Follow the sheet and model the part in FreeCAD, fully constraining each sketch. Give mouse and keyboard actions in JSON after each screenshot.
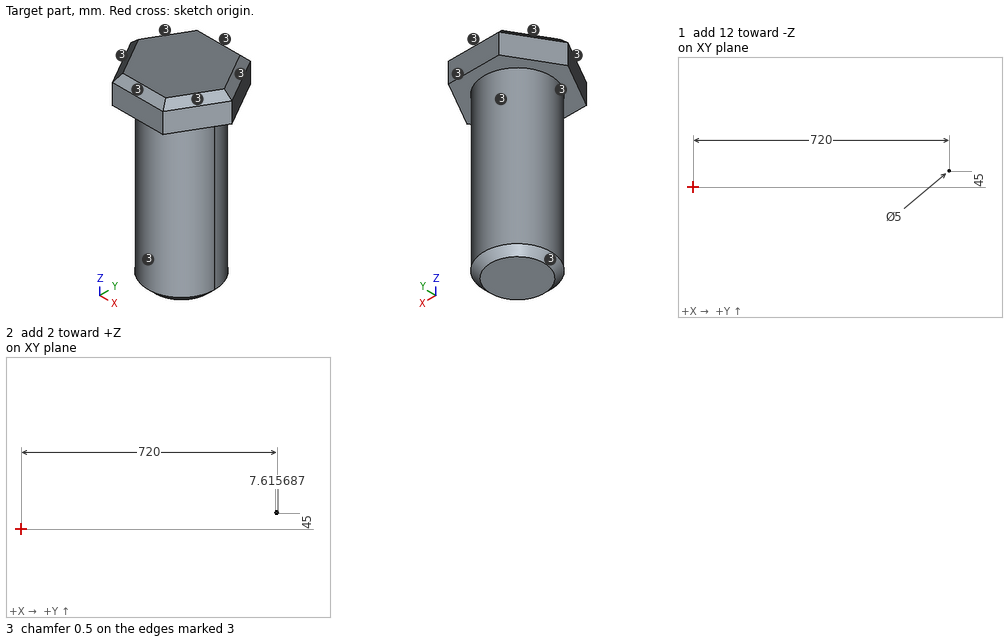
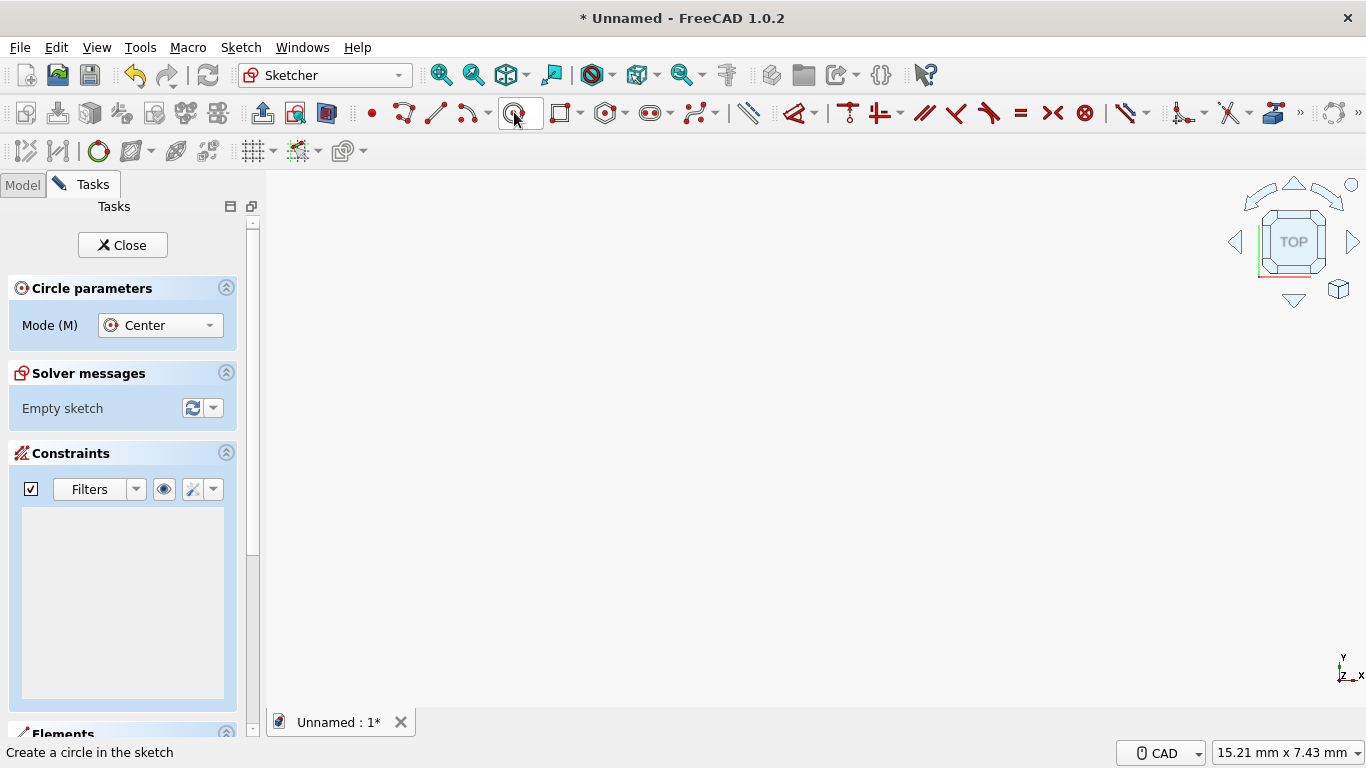
{"action": "left_click", "coordinate": [744, 437]}
{"action": "left_click", "coordinate": [871, 309]}
{"action": "key", "text": "Escape"}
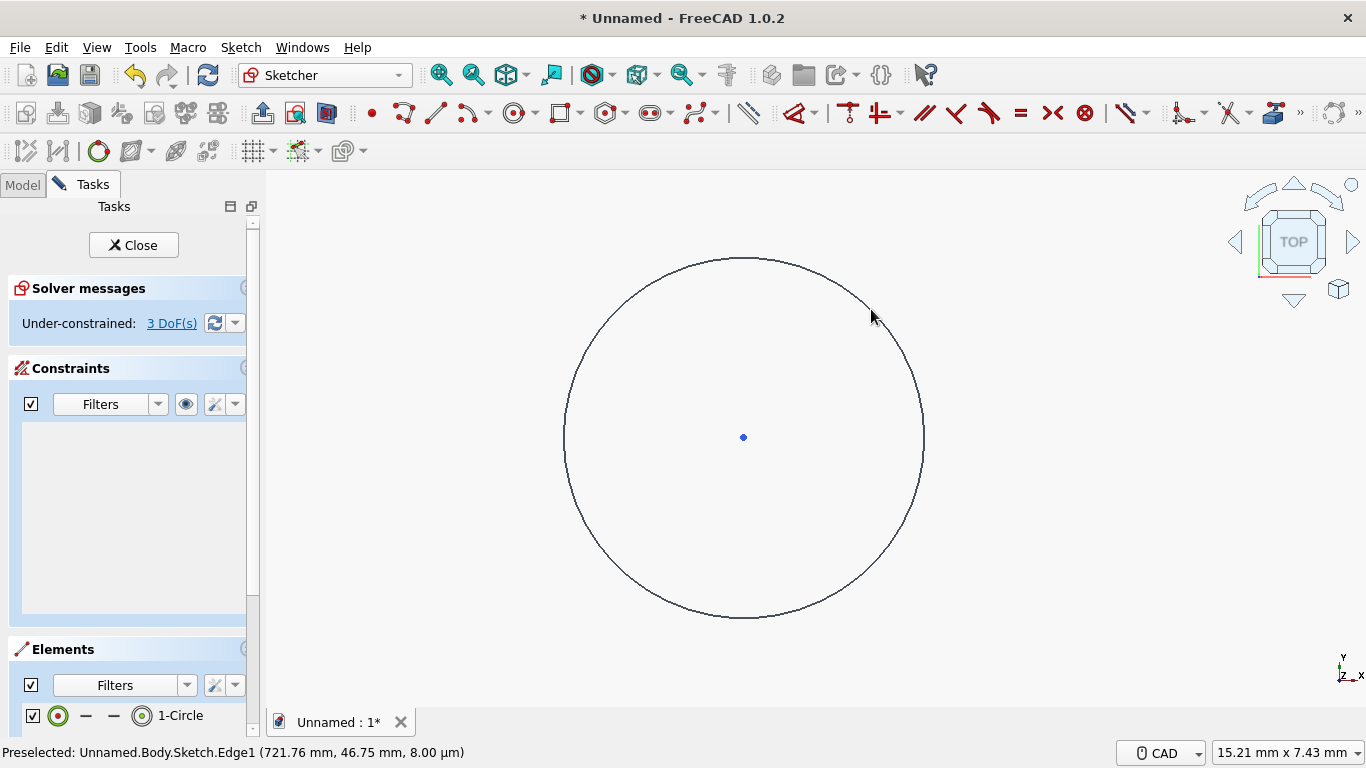
{"action": "key", "text": "d"}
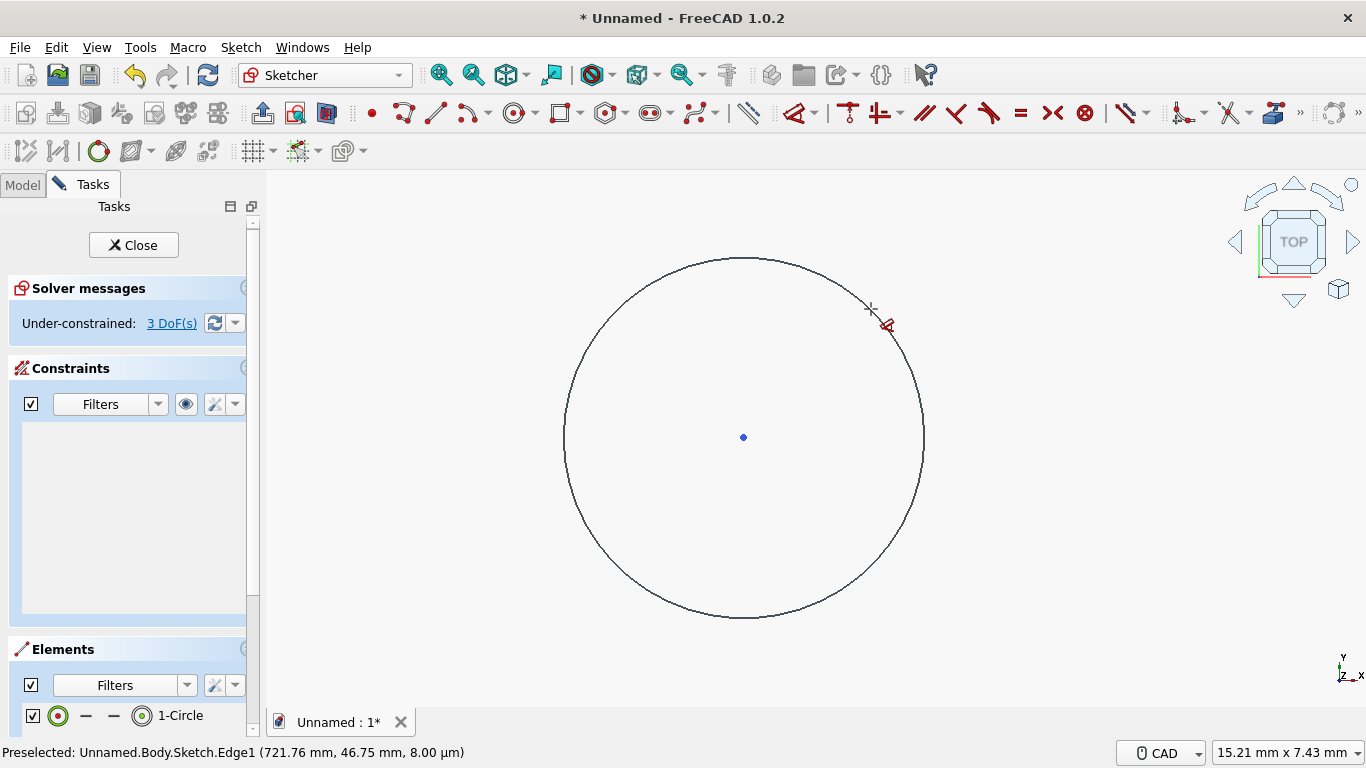
{"action": "left_click", "coordinate": [871, 310]}
{"action": "left_click", "coordinate": [894, 287]}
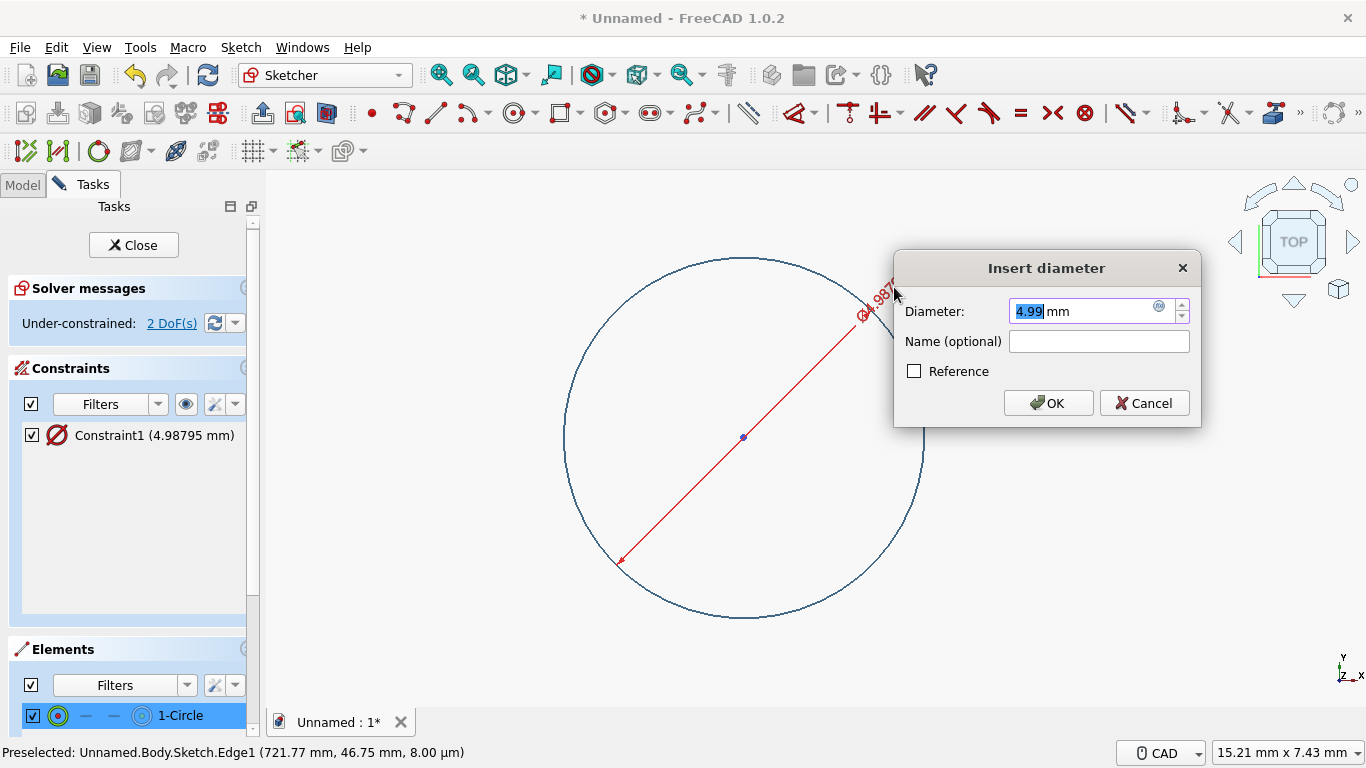
{"action": "type", "text": "5"}
{"action": "key", "text": "Return"}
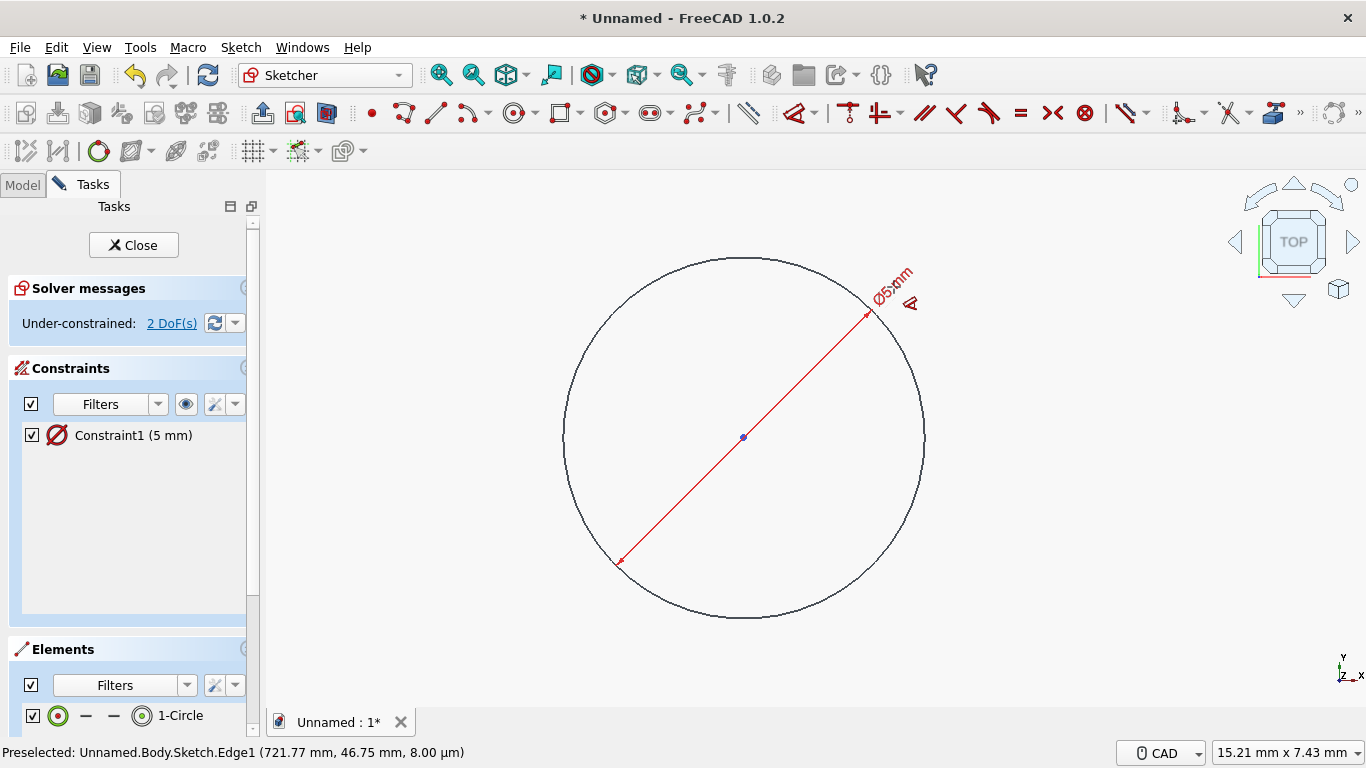
{"action": "left_click", "coordinate": [744, 438]}
{"action": "left_click", "coordinate": [778, 558]}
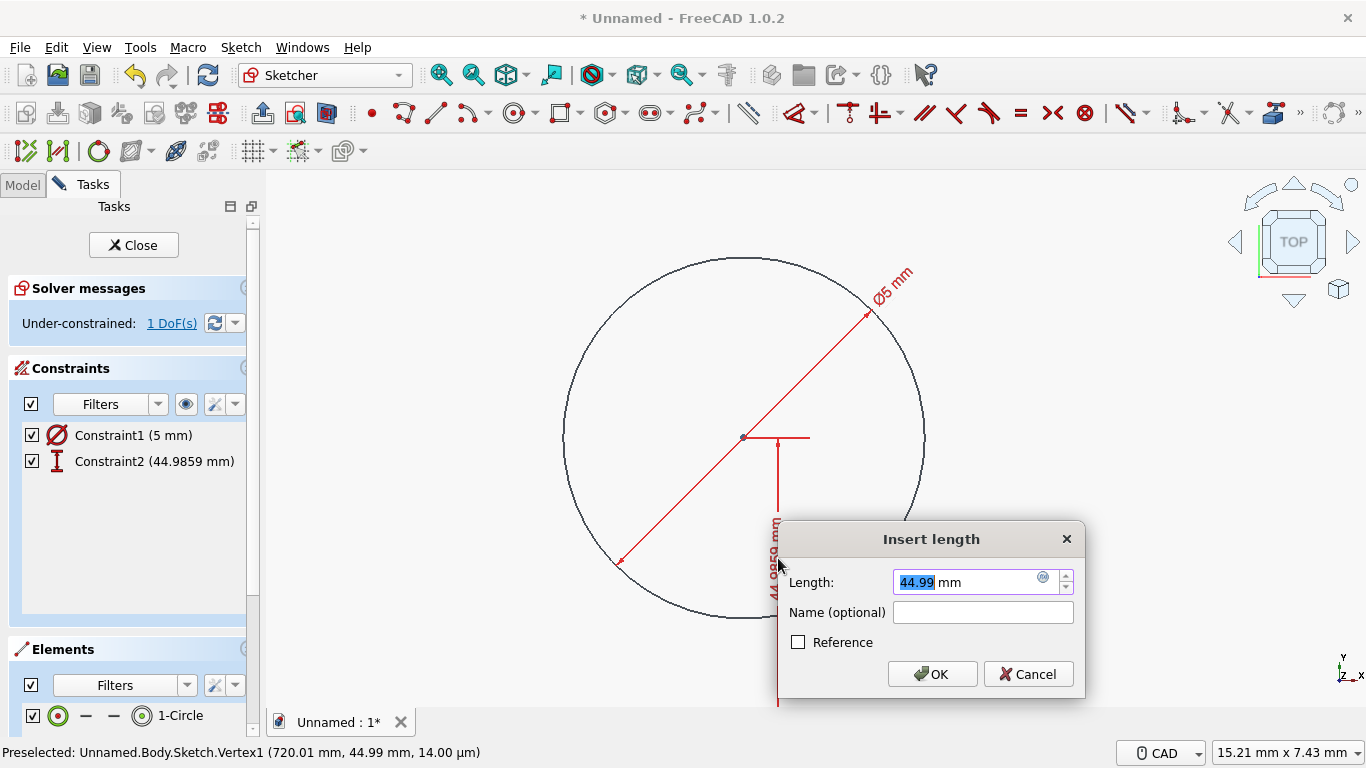
{"action": "type", "text": "45"}
{"action": "key", "text": "Return"}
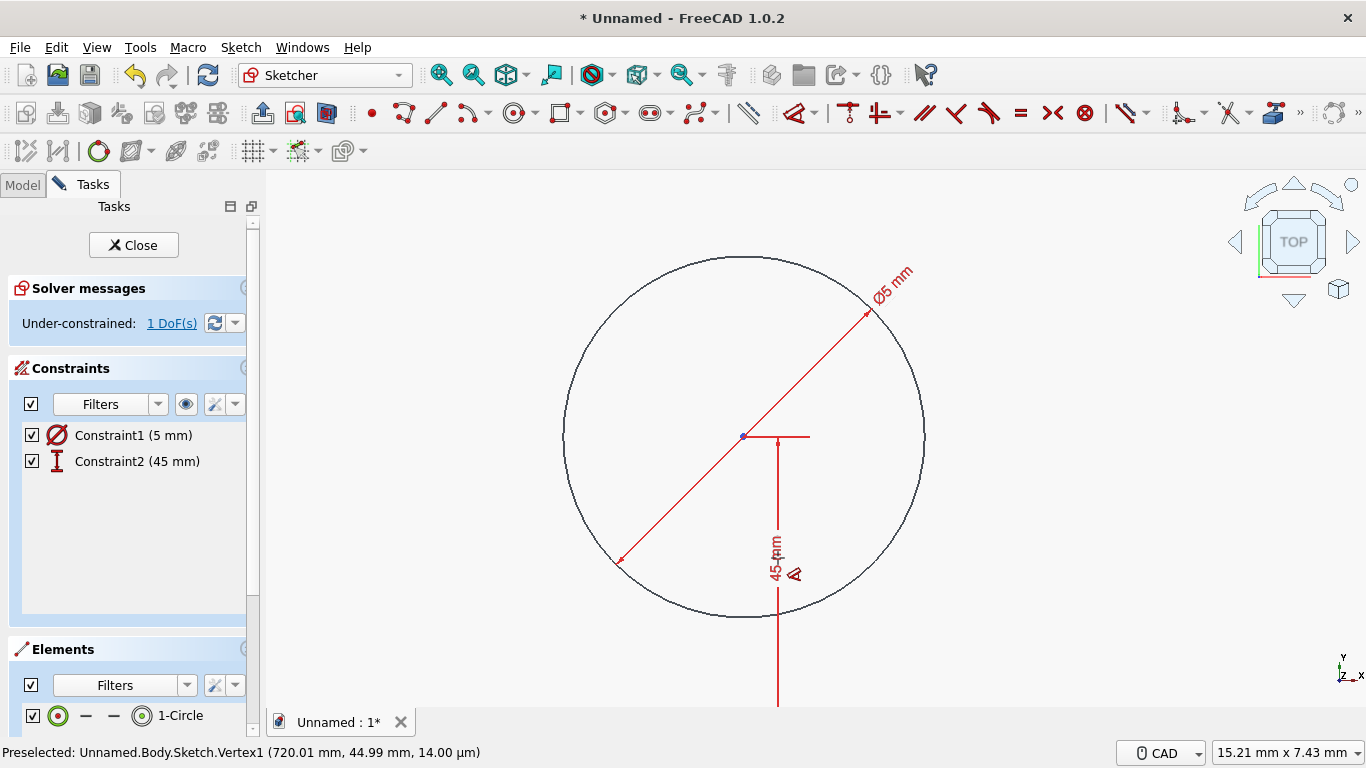
{"action": "left_click", "coordinate": [744, 437]}
{"action": "left_click", "coordinate": [519, 403]}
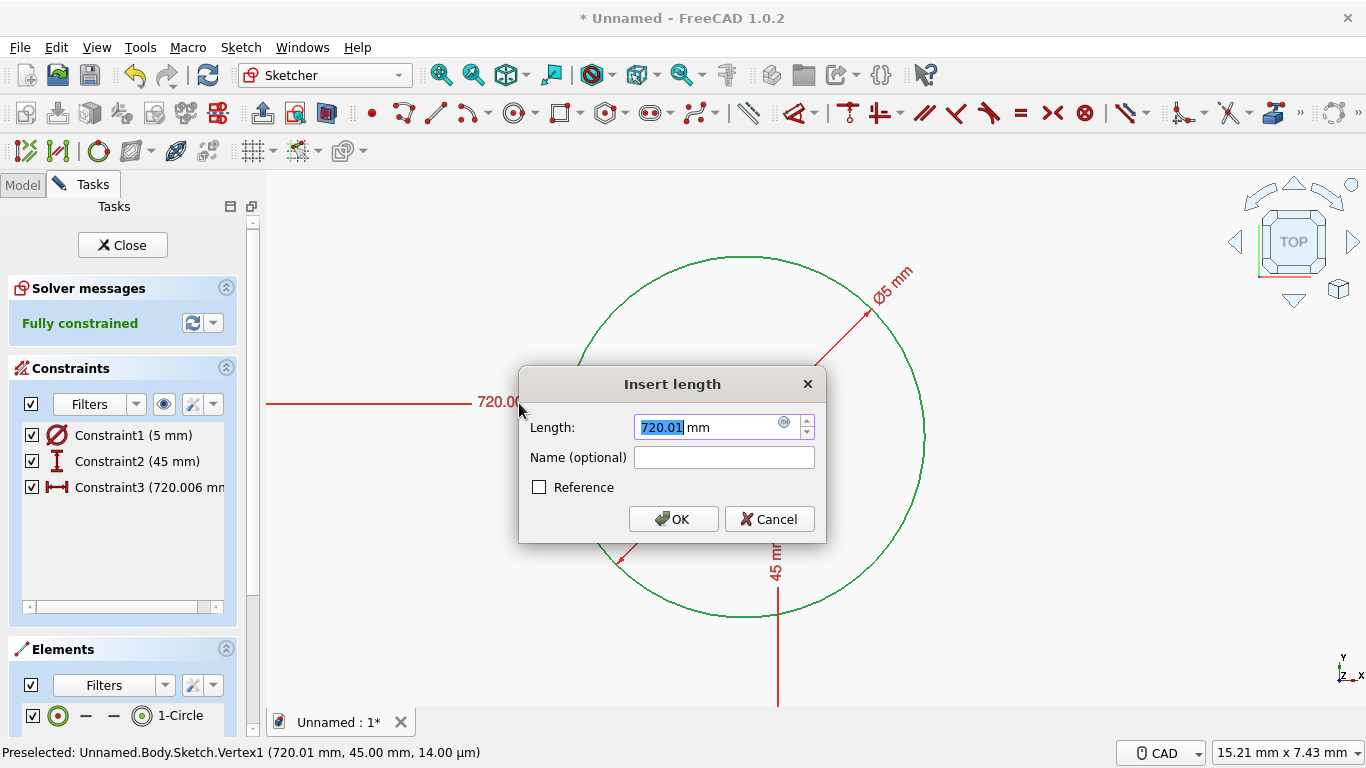
{"action": "type", "text": "720"}
{"action": "key", "text": "Return"}
{"action": "key", "text": "Escape"}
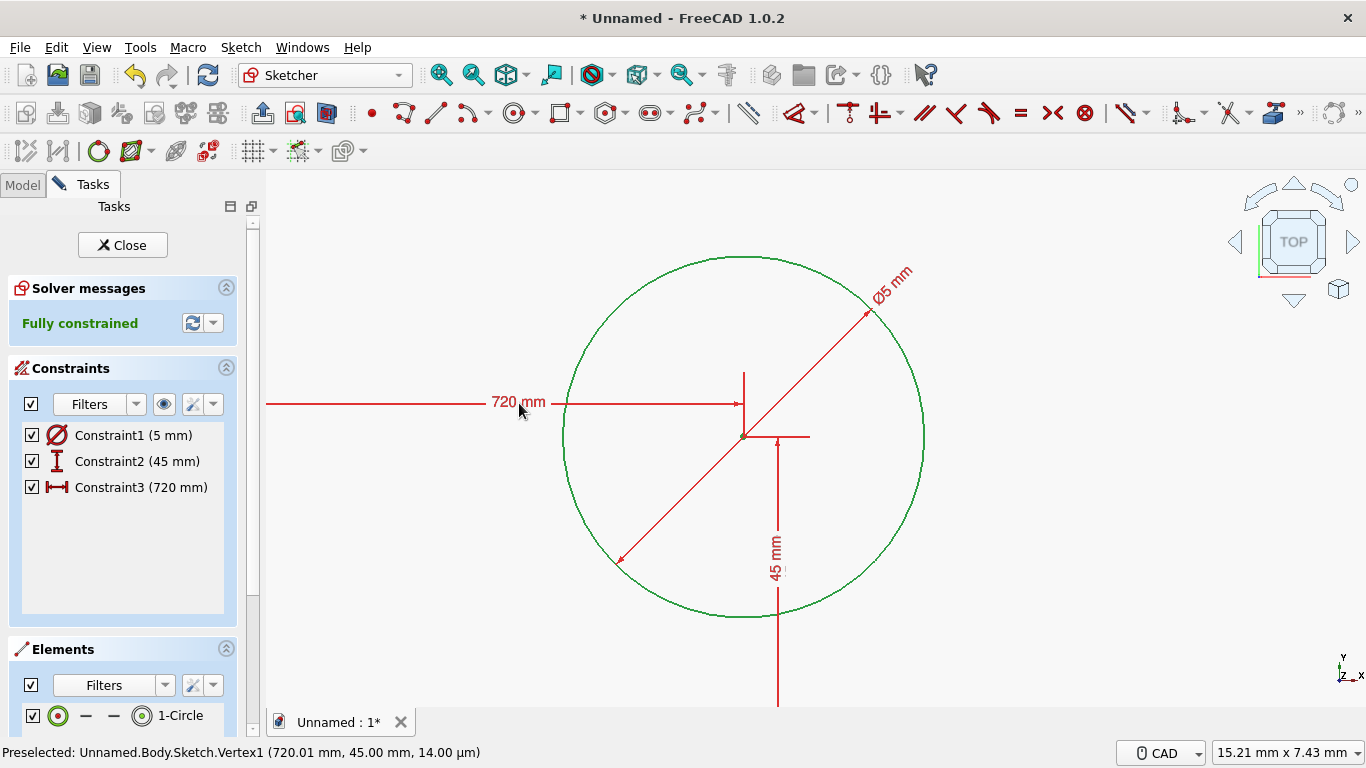
{"action": "left_click", "coordinate": [123, 245]}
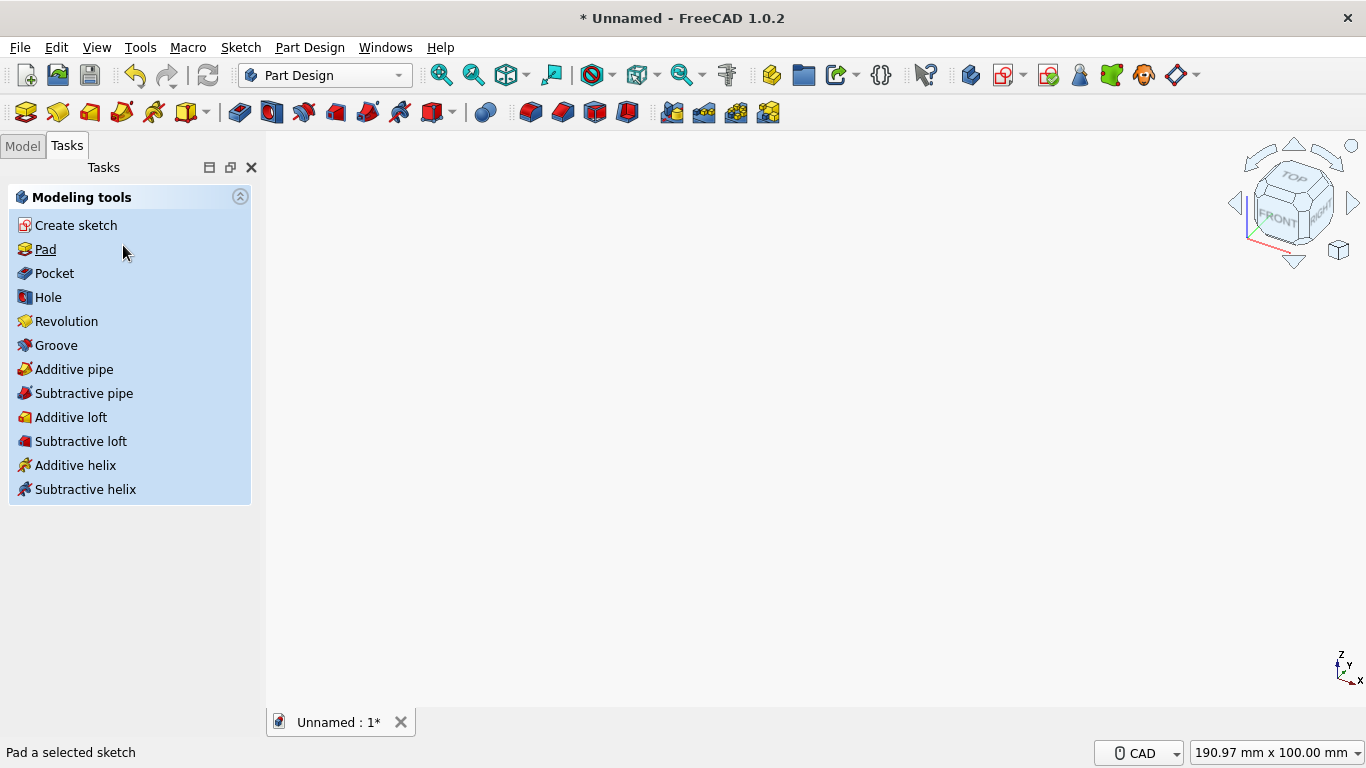
{"action": "left_click", "coordinate": [26, 112]}